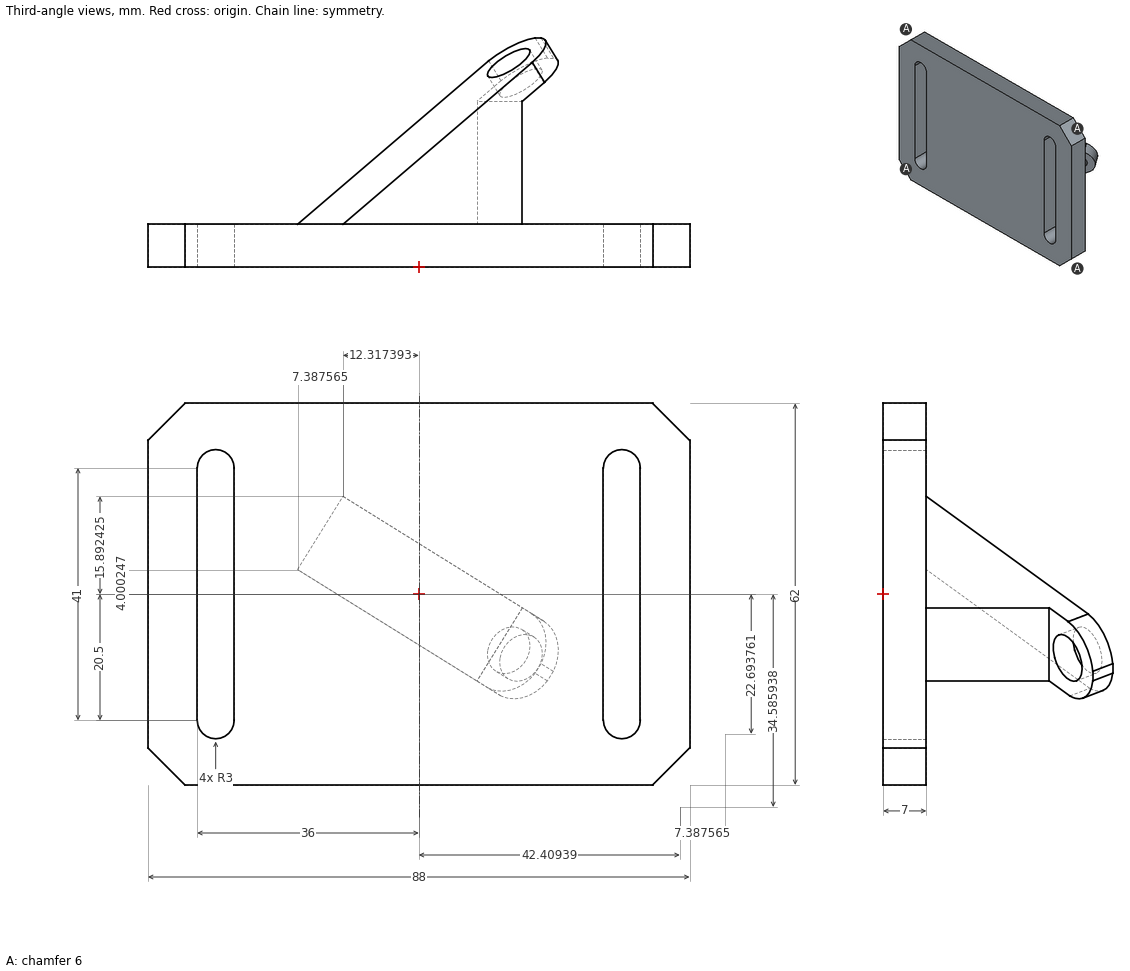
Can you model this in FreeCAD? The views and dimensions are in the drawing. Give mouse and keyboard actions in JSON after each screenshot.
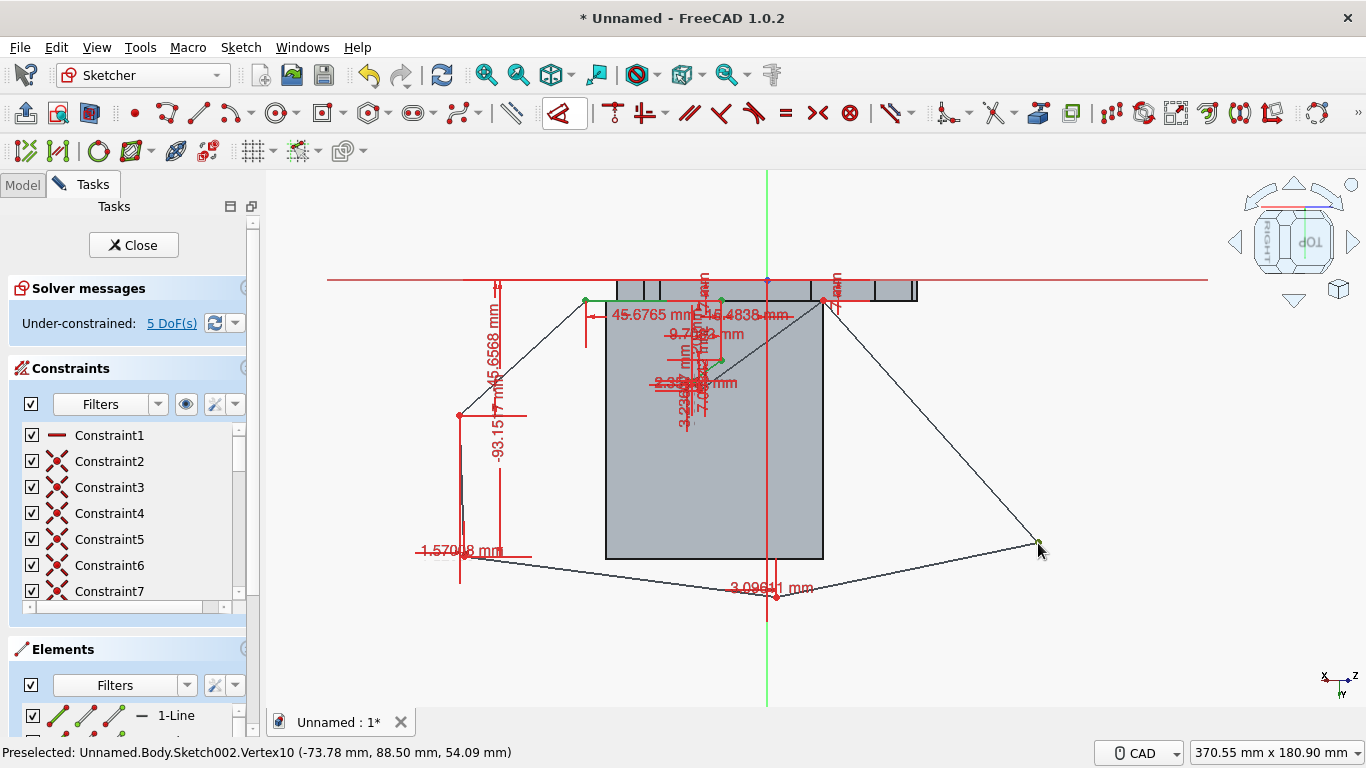
{"action": "left_click", "coordinate": [582, 114]}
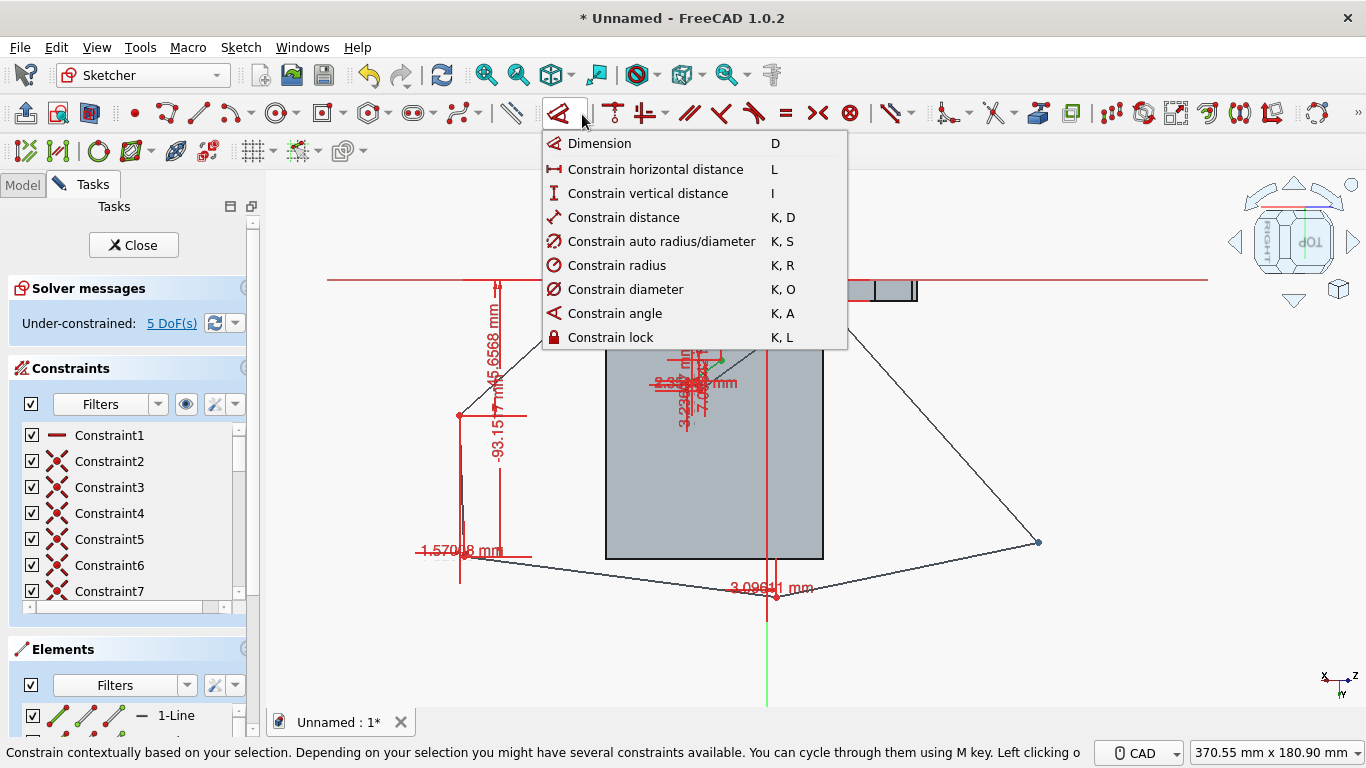
{"action": "left_click", "coordinate": [695, 169]}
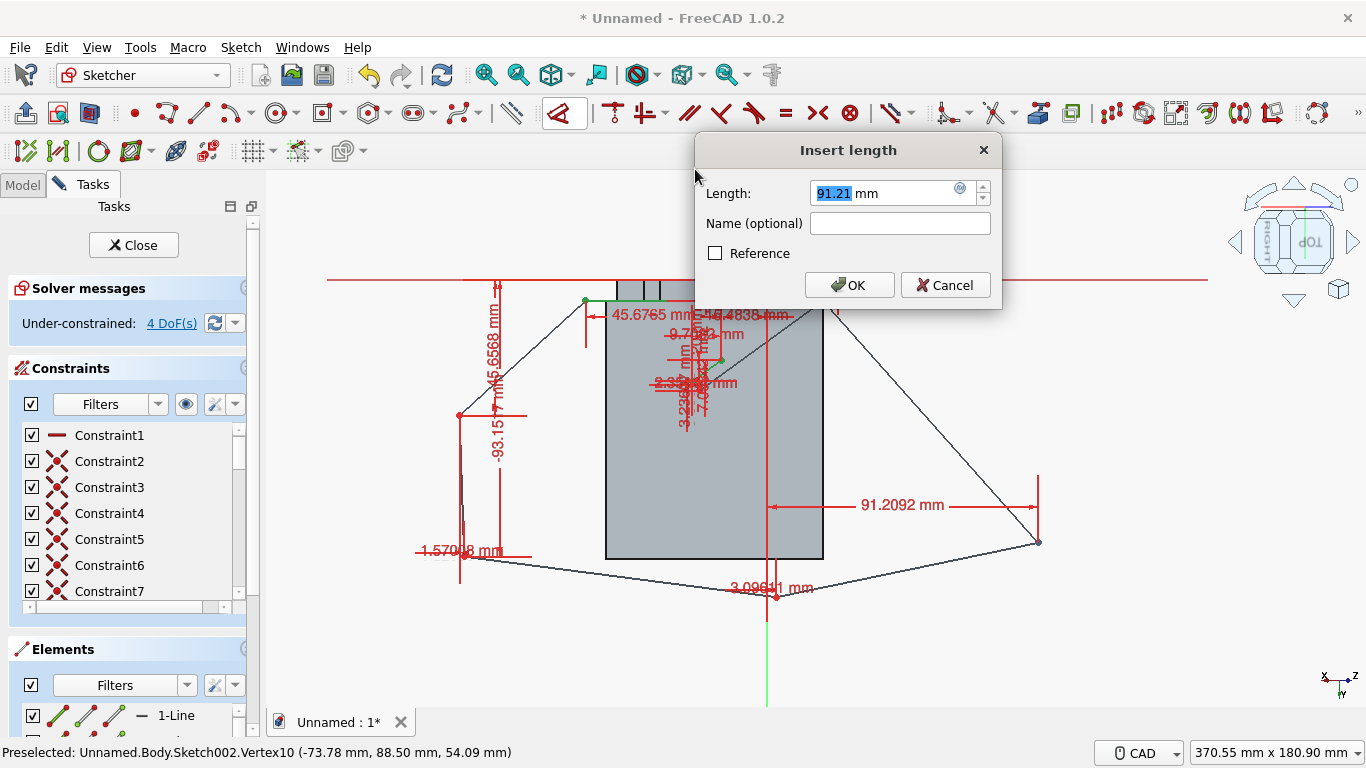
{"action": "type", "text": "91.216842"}
{"action": "key", "text": "Return"}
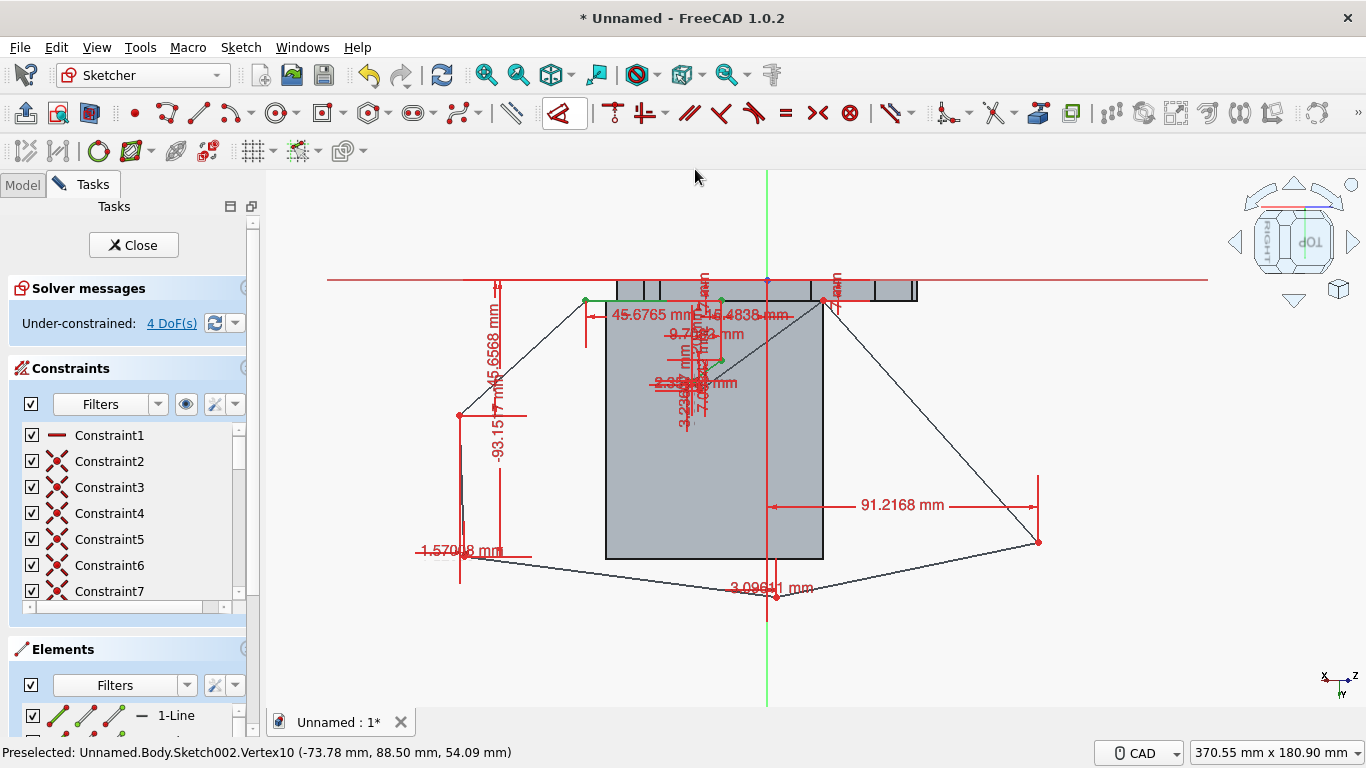
{"action": "left_click", "coordinate": [1038, 543]}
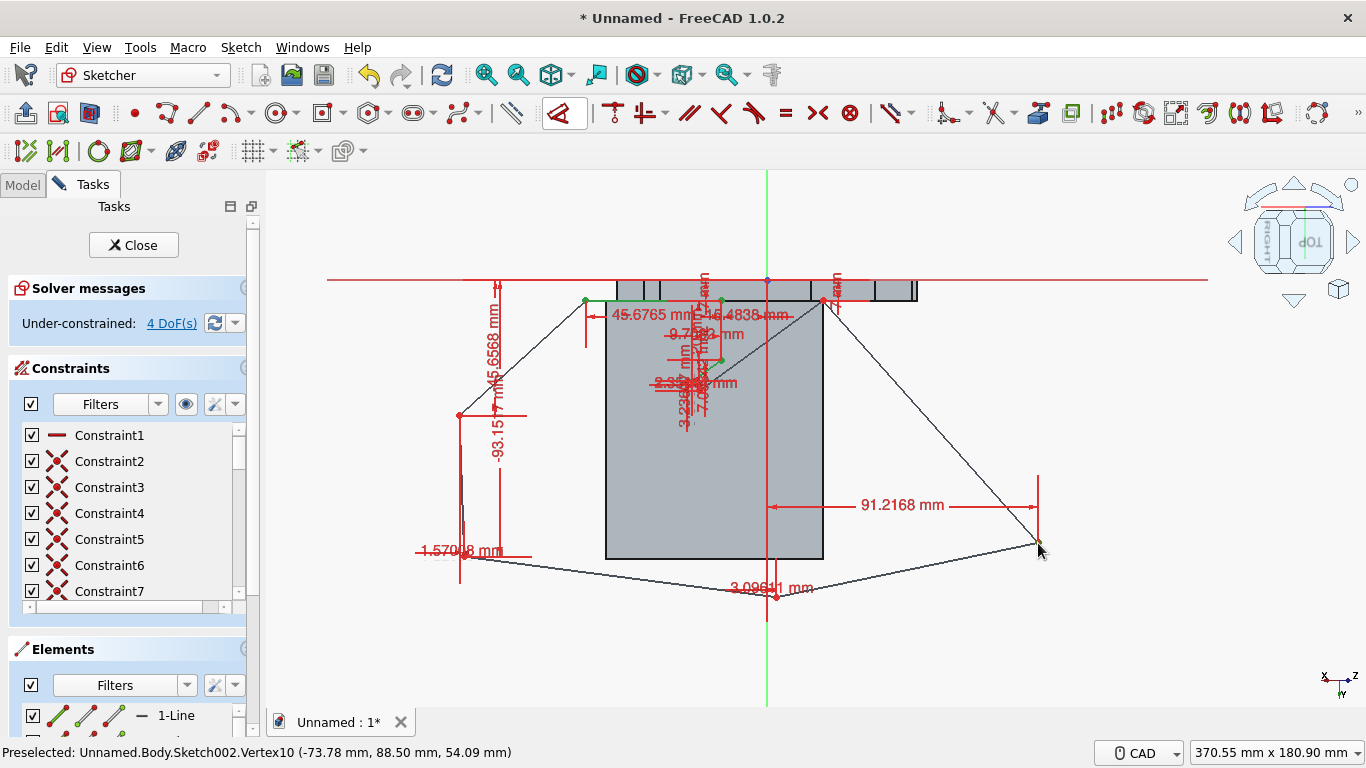
{"action": "left_click", "coordinate": [582, 114]}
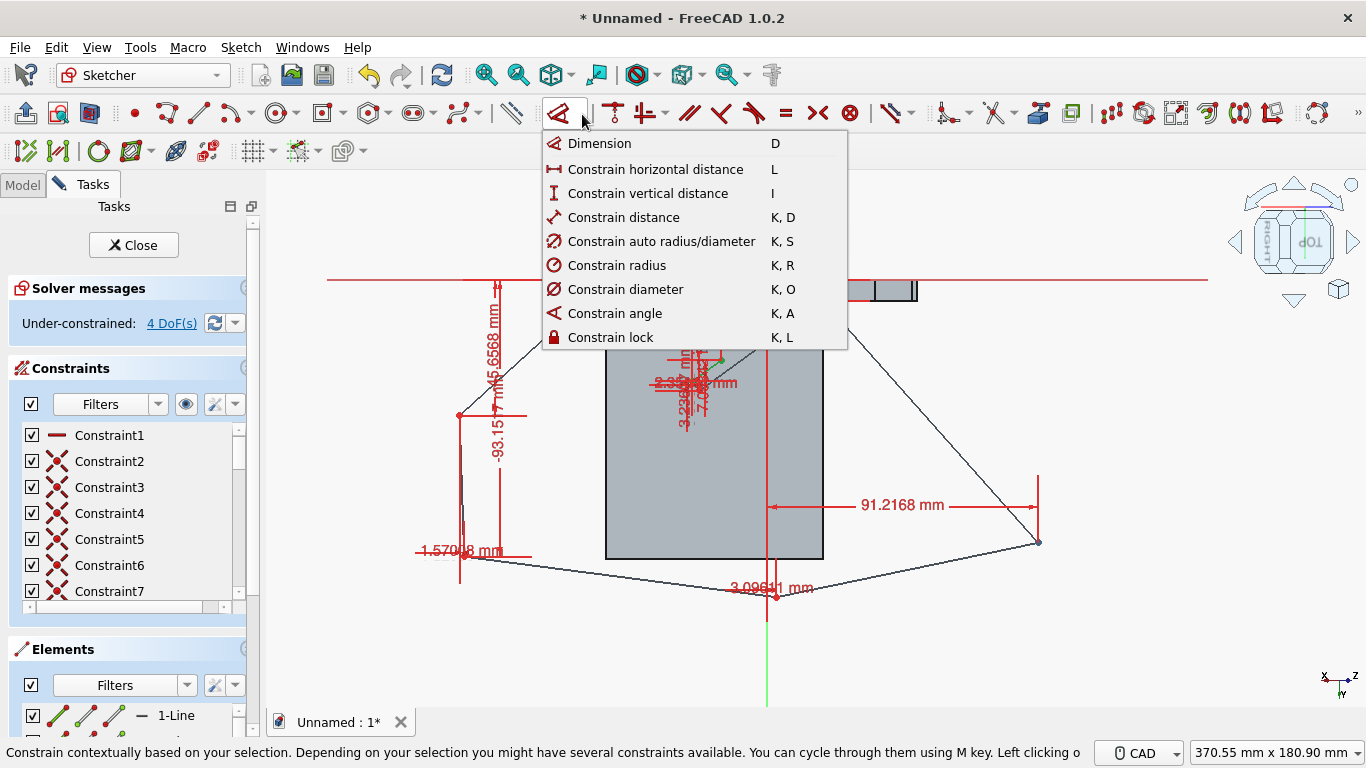
{"action": "left_click", "coordinate": [695, 193]}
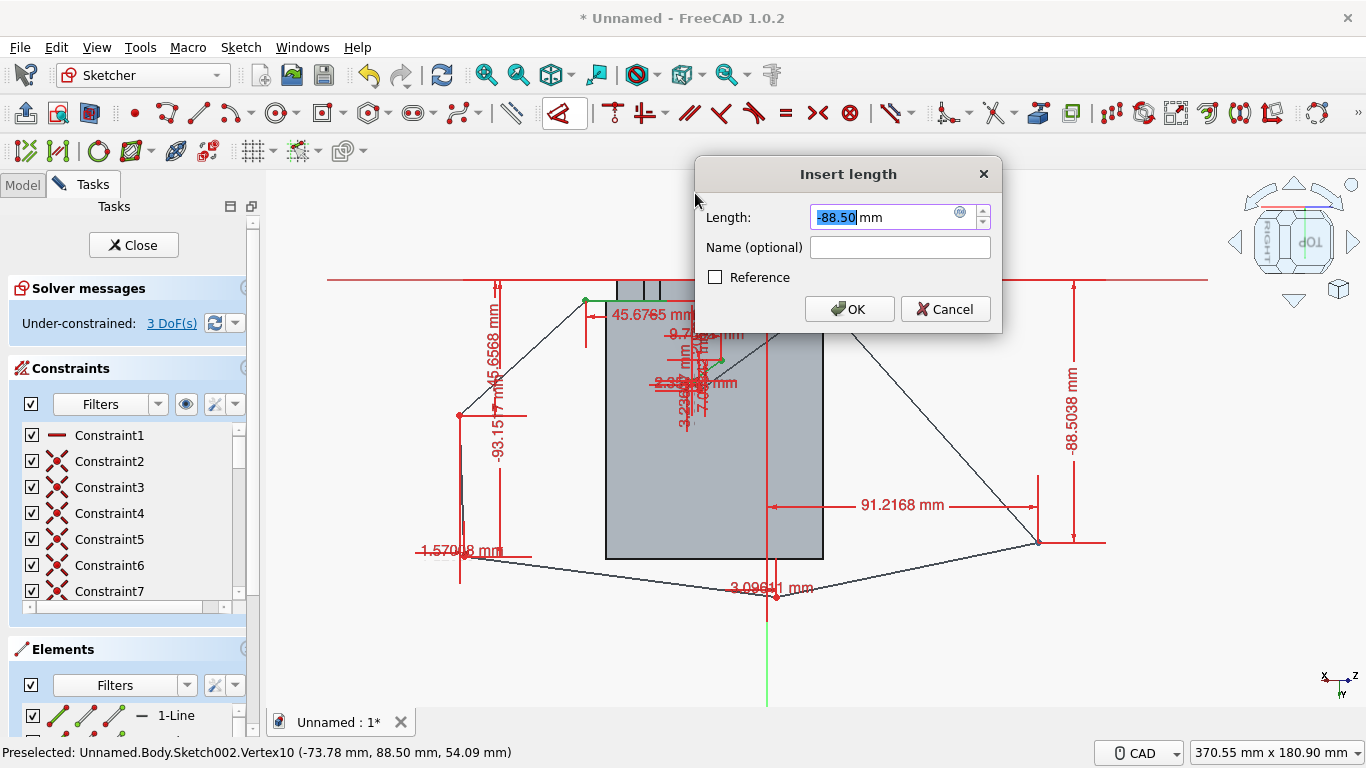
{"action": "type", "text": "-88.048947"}
{"action": "key", "text": "Return"}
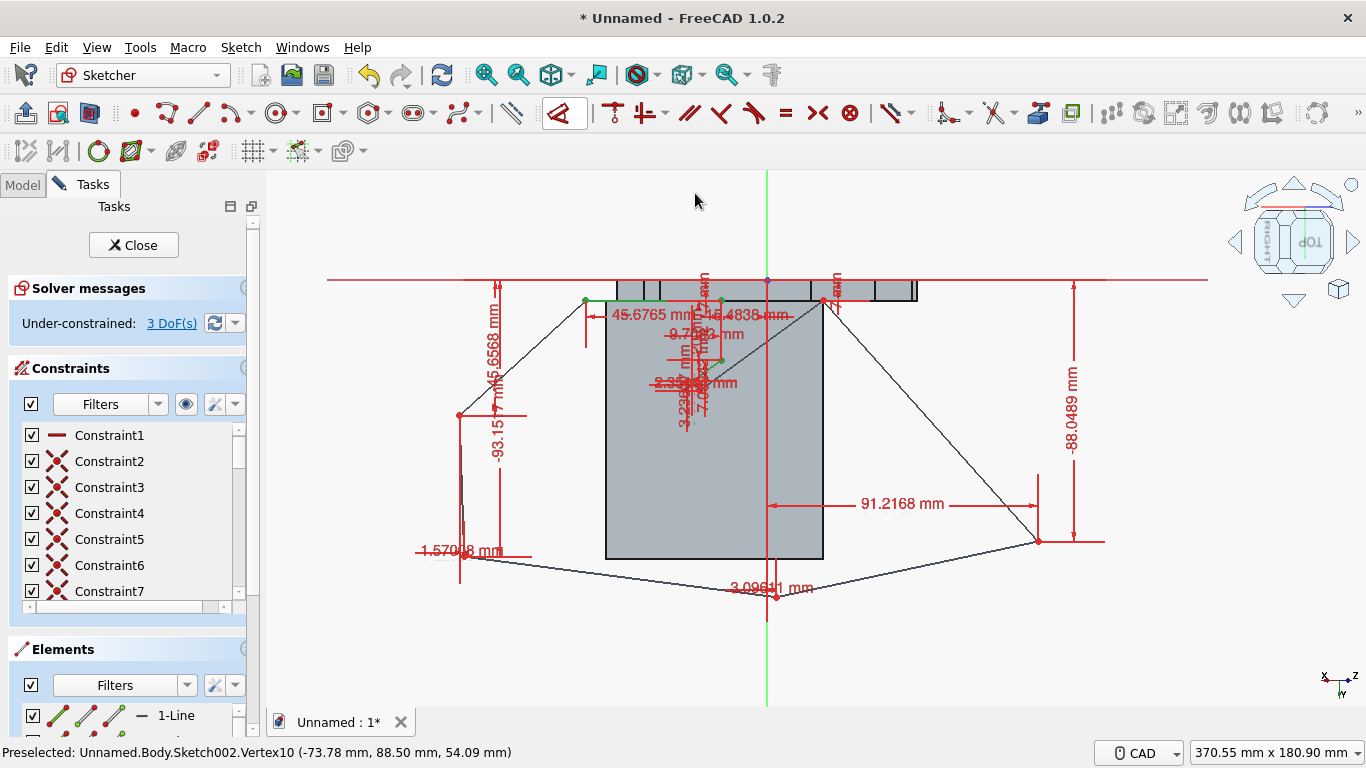
{"action": "left_click", "coordinate": [823, 301]}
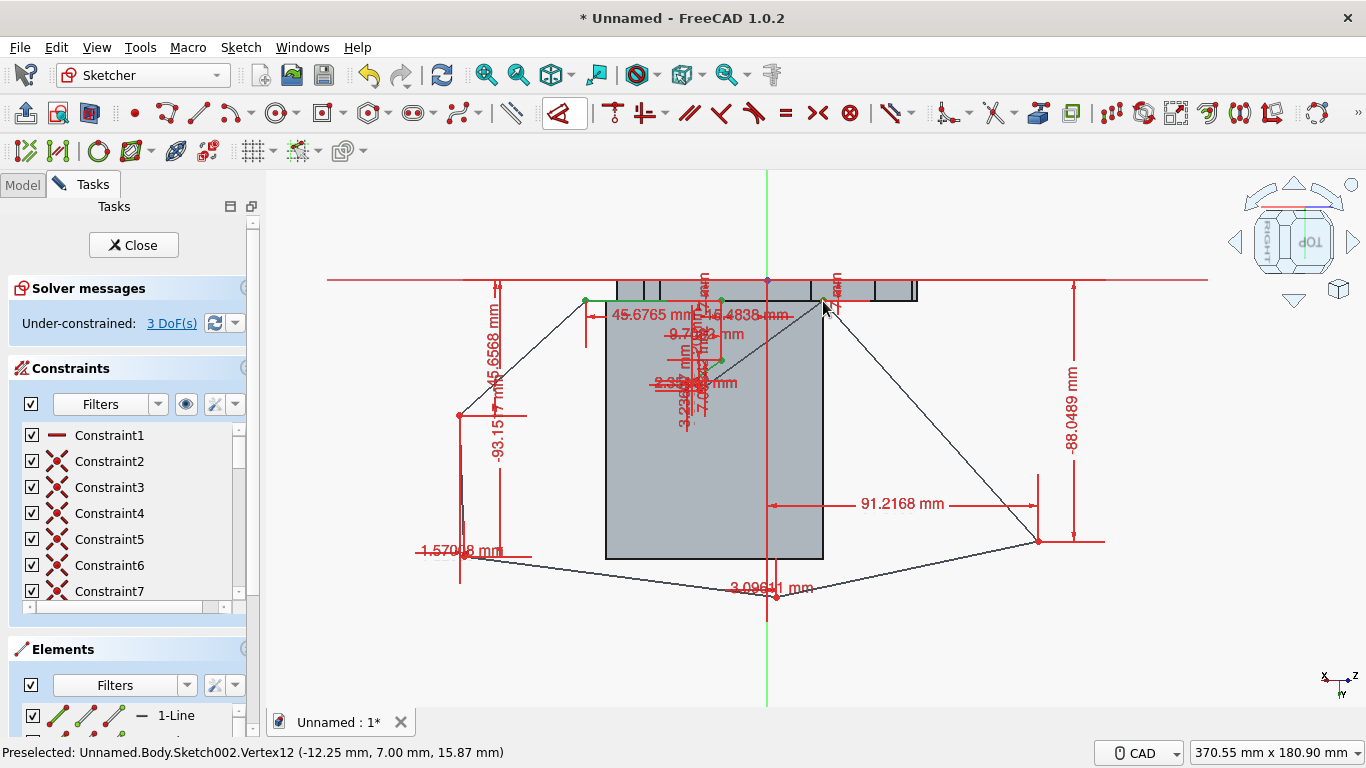
{"action": "key", "text": "l"}